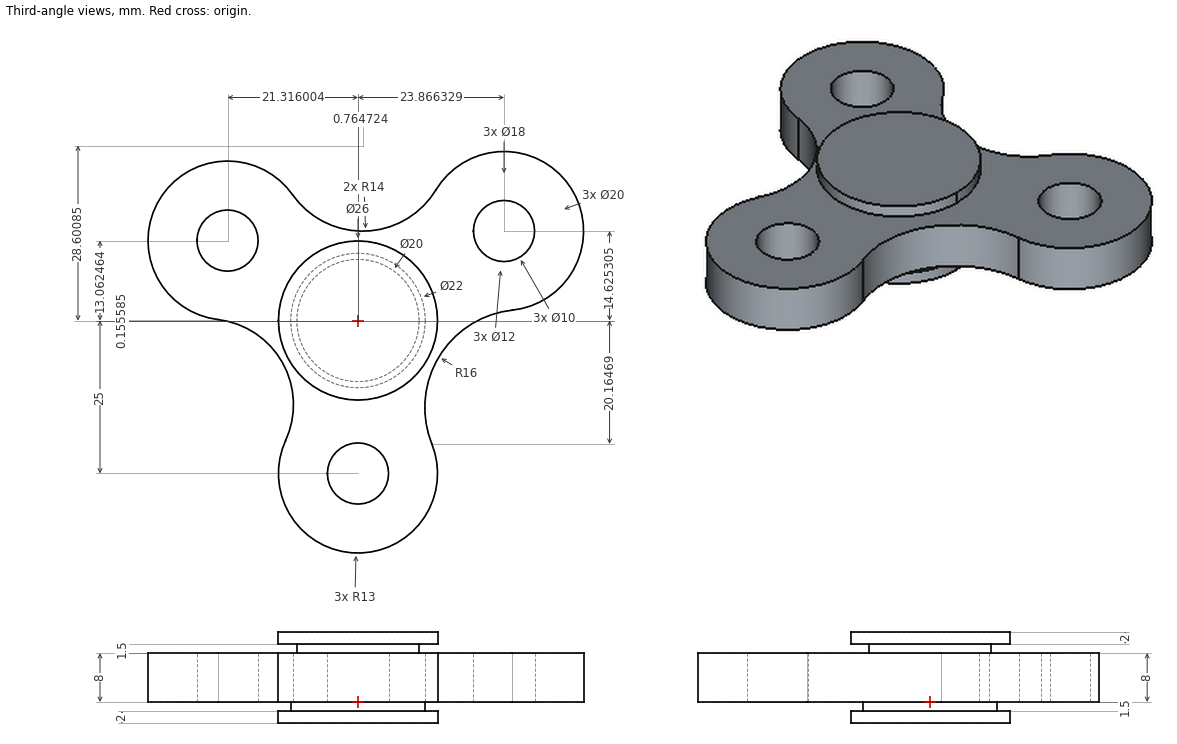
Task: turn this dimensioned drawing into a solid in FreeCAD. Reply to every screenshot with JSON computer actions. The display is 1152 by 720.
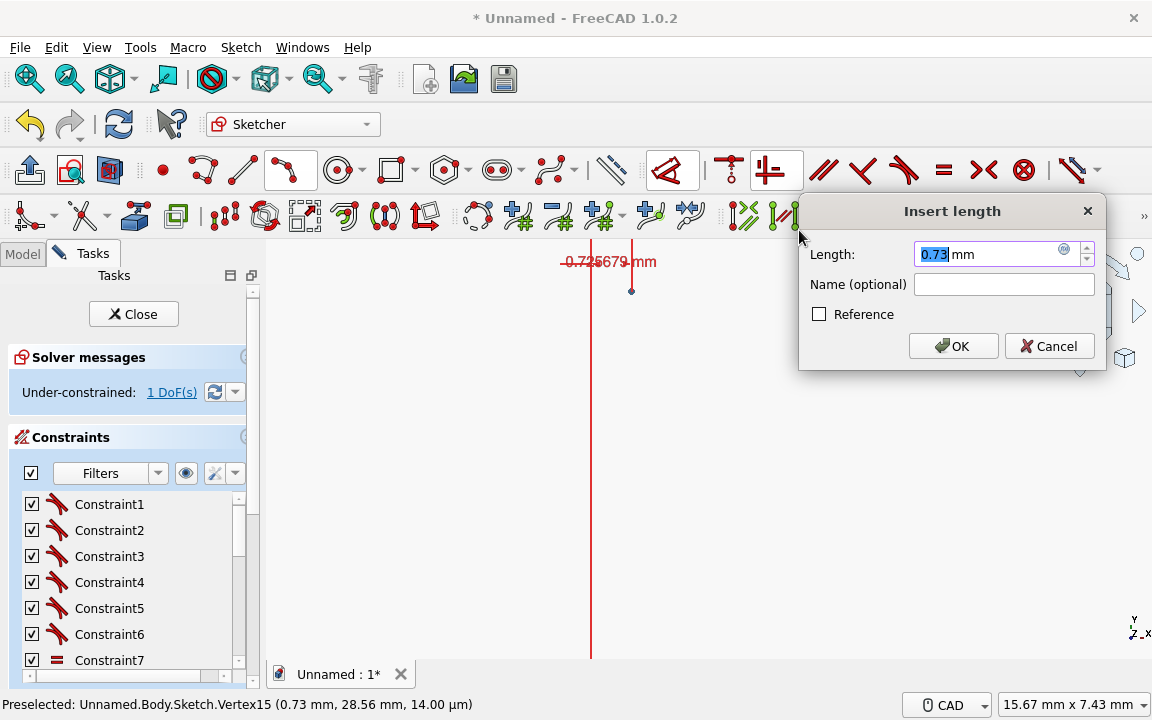
{"action": "type", "text": "0.764724"}
{"action": "key", "text": "Return"}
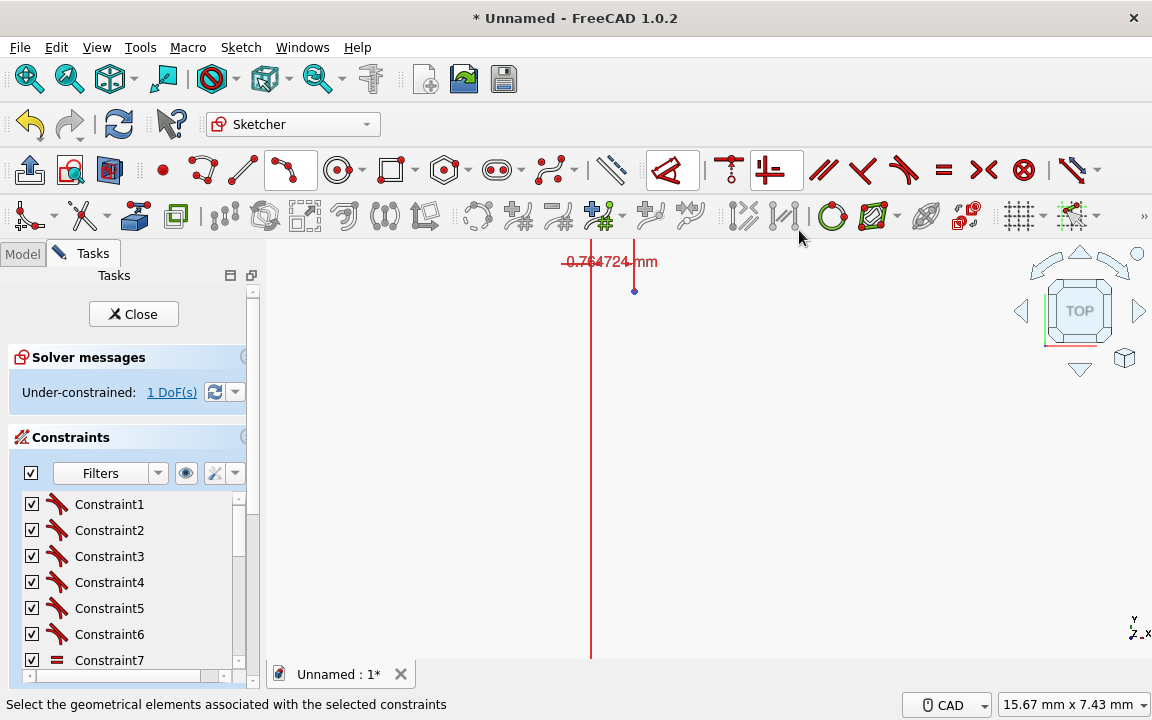
{"action": "scroll", "coordinate": [639, 295], "scroll_direction": "down", "scroll_amount": 13}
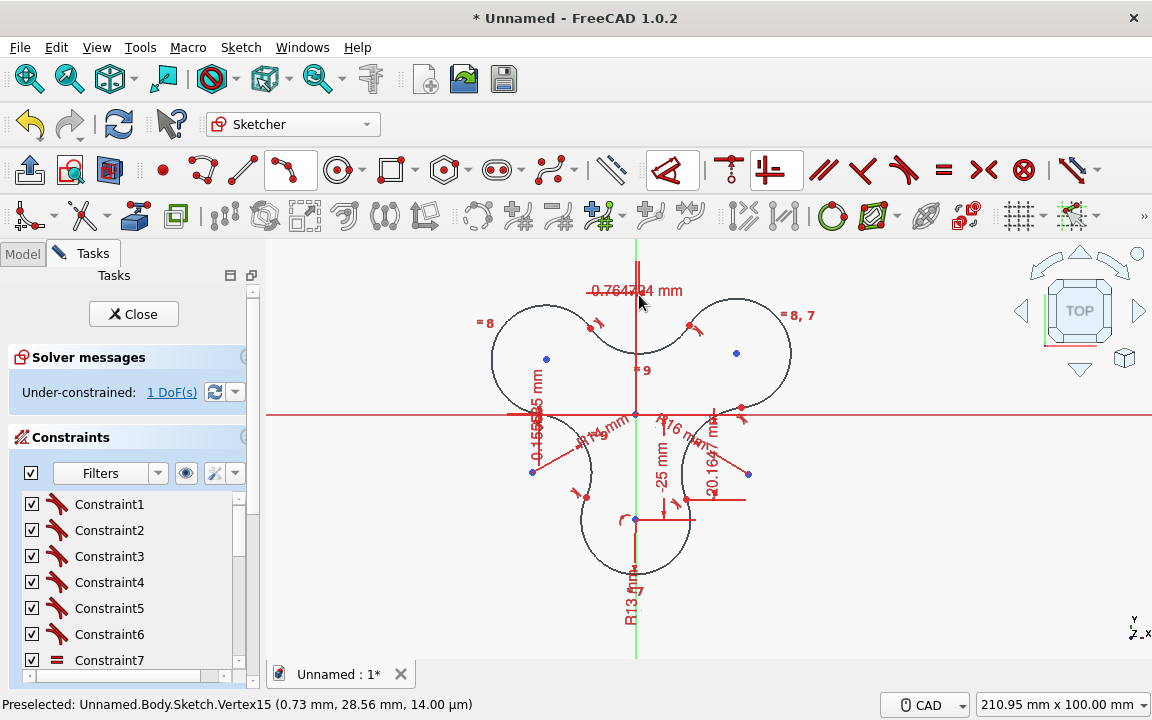
{"action": "left_click", "coordinate": [639, 295]}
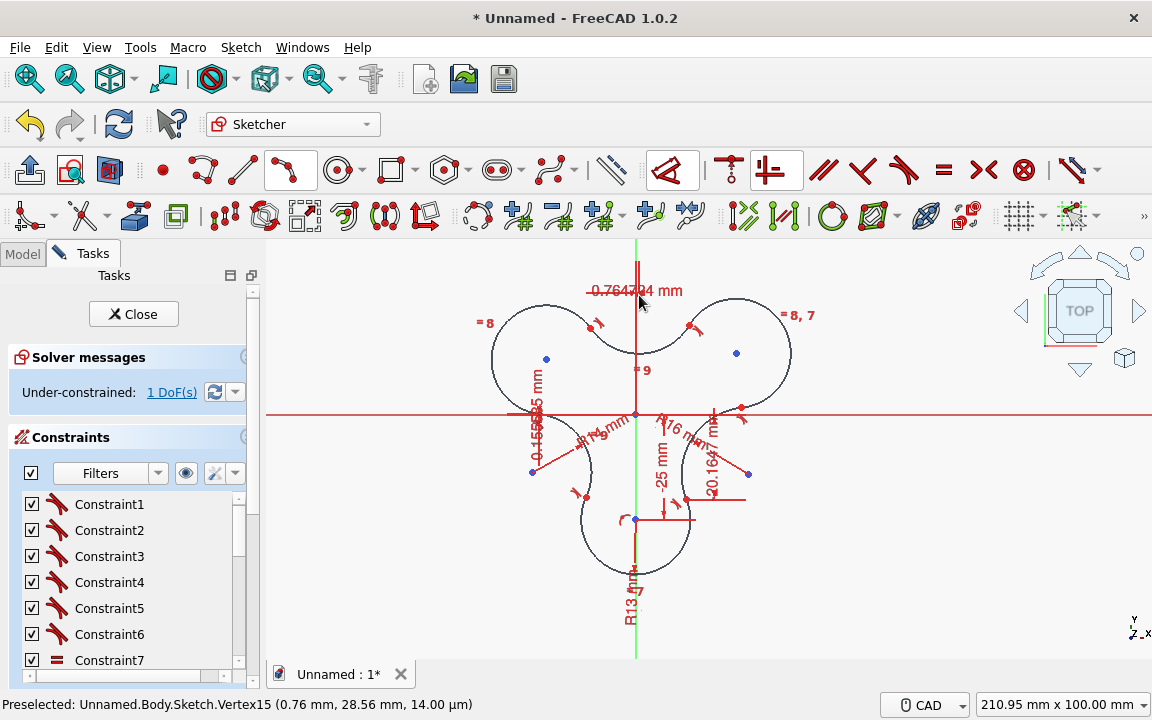
{"action": "key", "text": "i"}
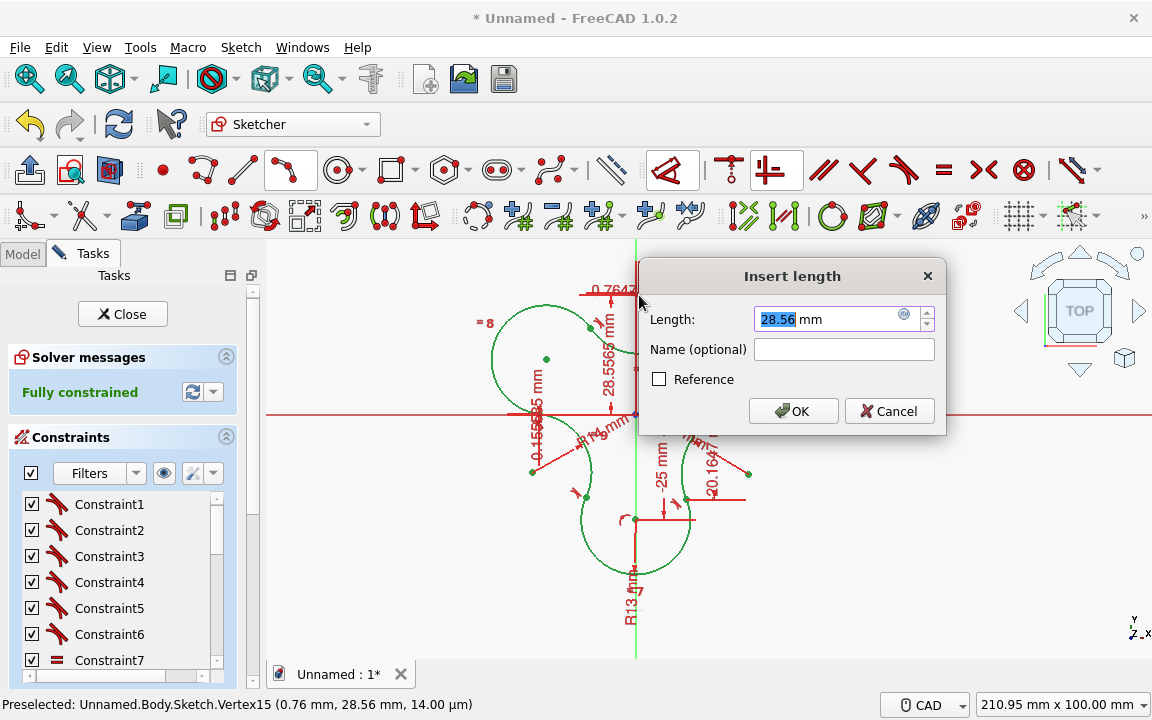
{"action": "type", "text": "28.60085"}
{"action": "key", "text": "Return"}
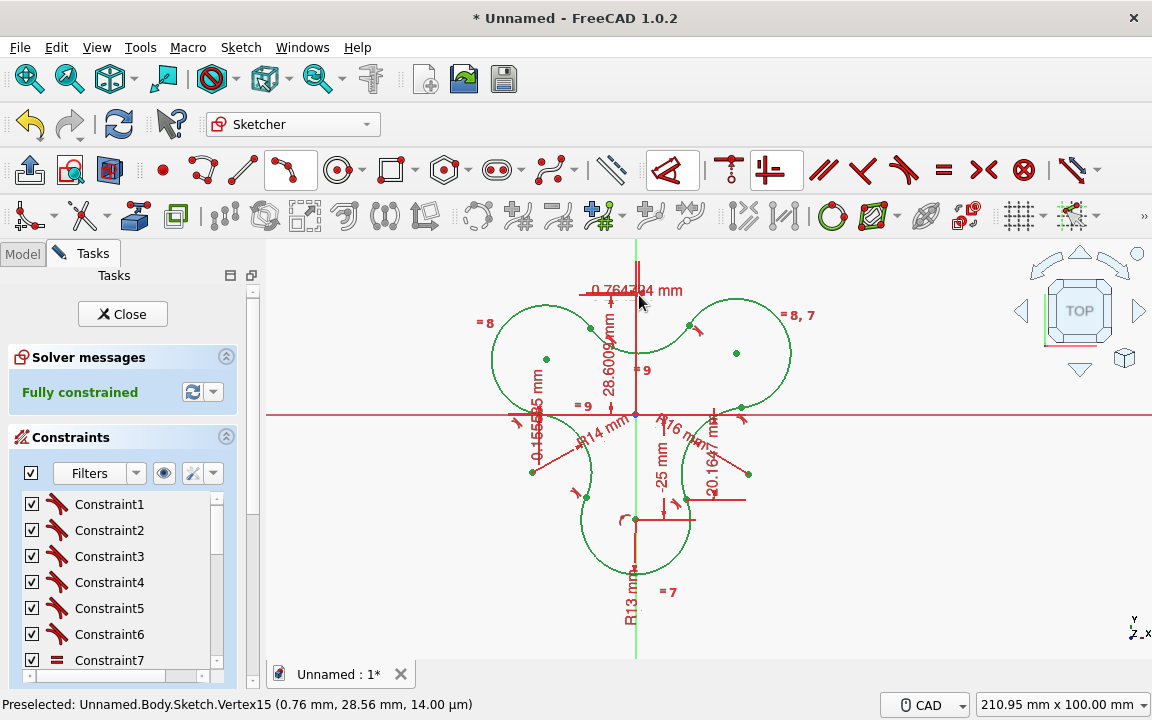
{"action": "left_click", "coordinate": [123, 314]}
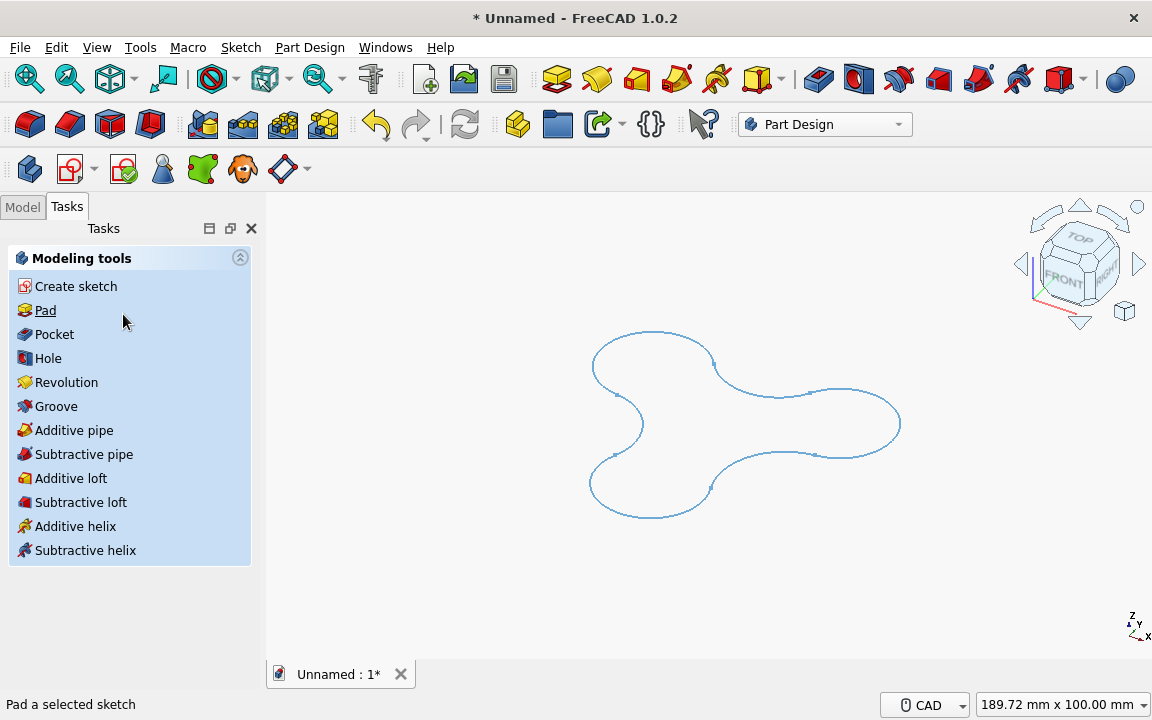
{"action": "left_click", "coordinate": [558, 80]}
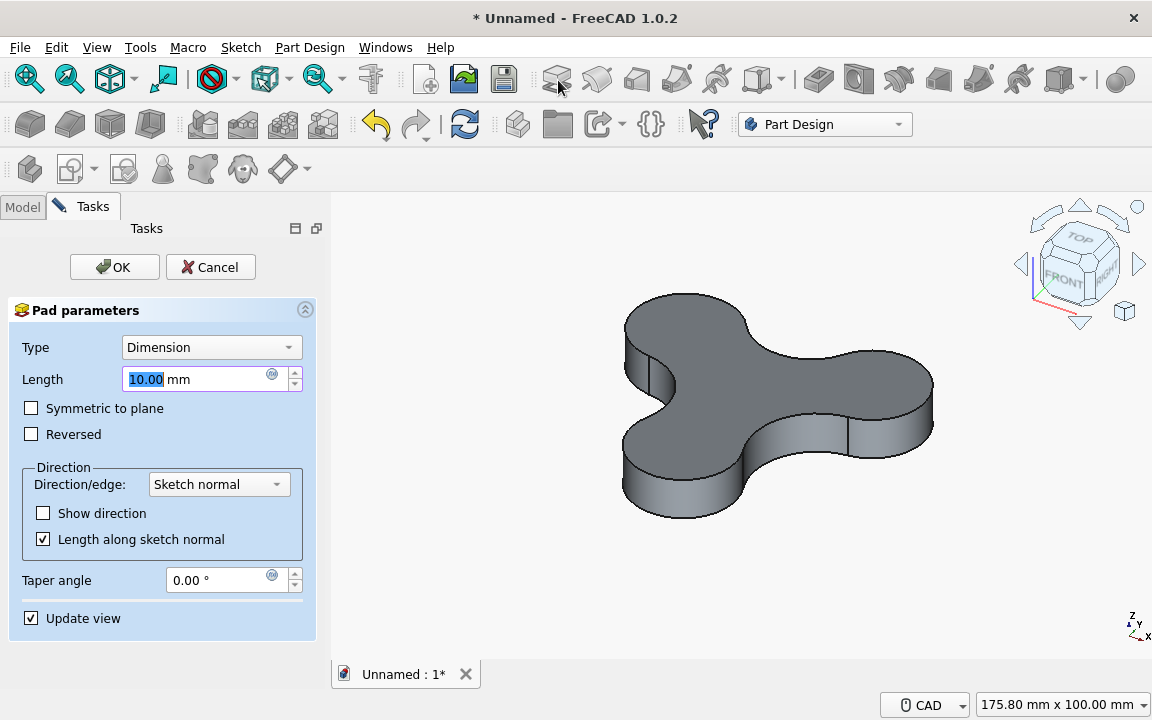
{"action": "type", "text": "8"}
{"action": "key", "text": "Tab"}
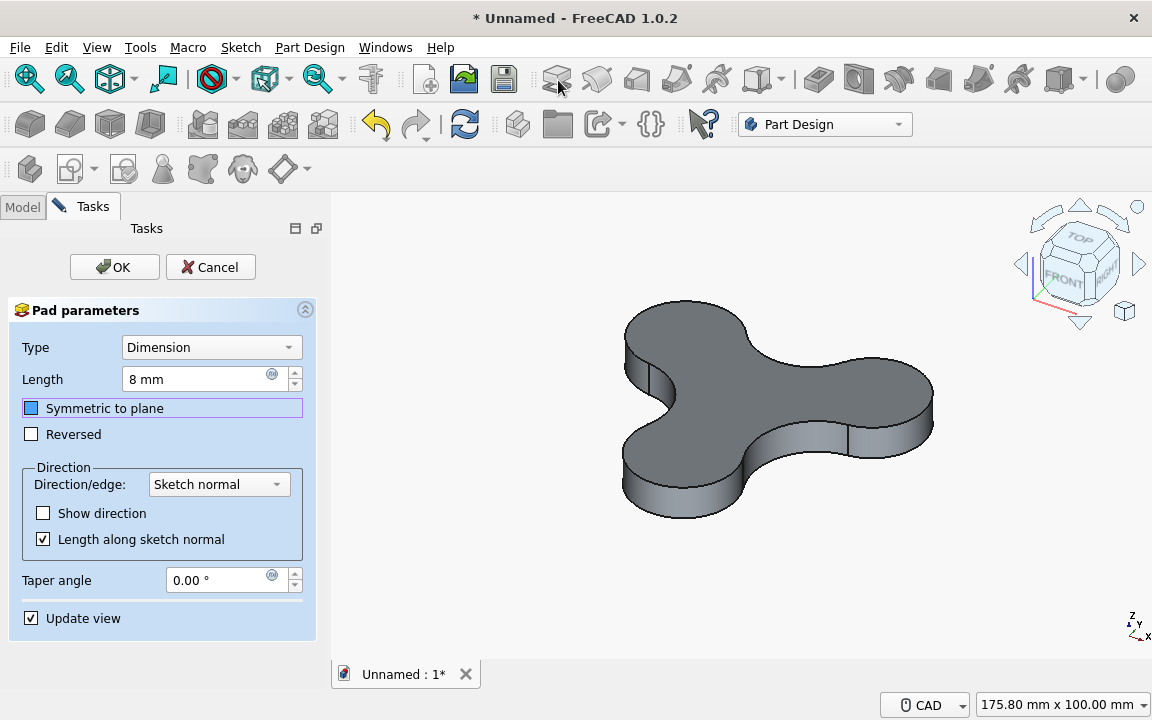
{"action": "left_click", "coordinate": [115, 267]}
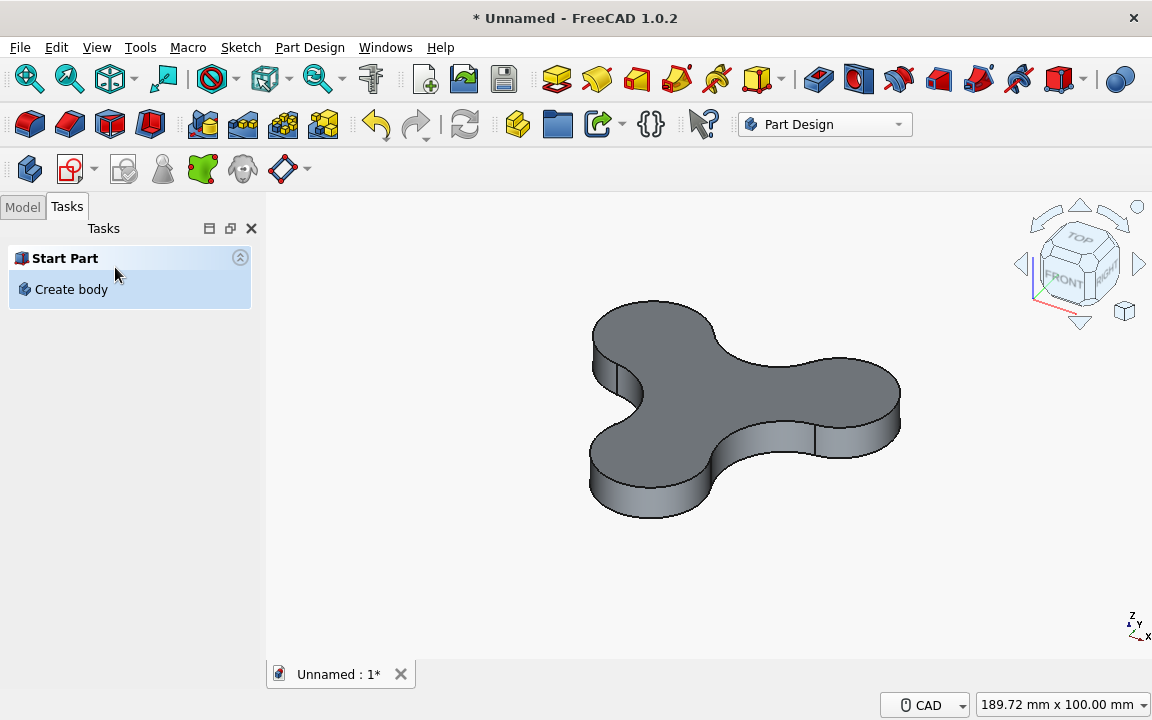
{"action": "left_click", "coordinate": [828, 391]}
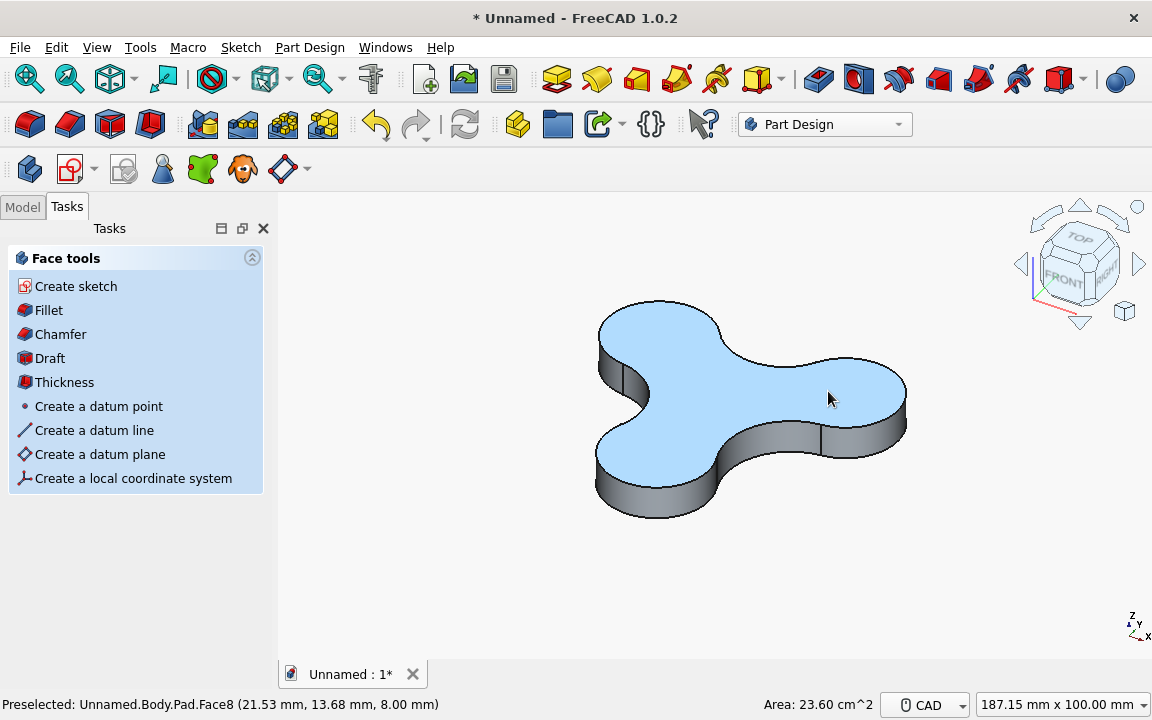
{"action": "left_click", "coordinate": [70, 170]}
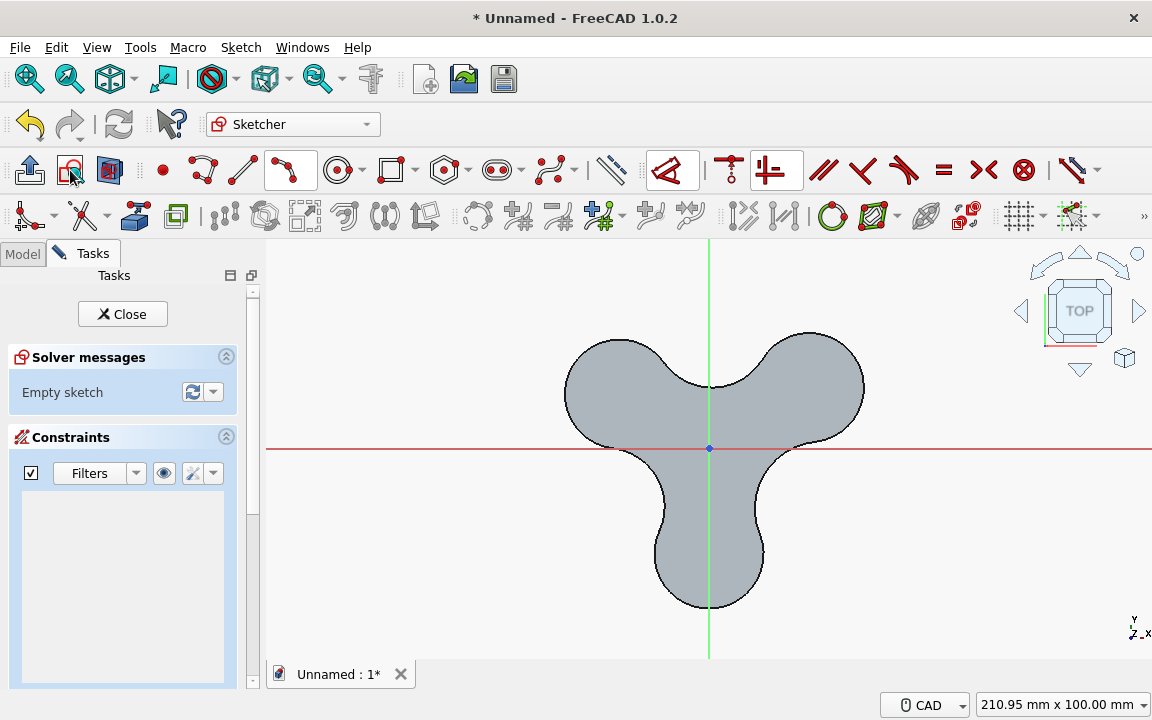
{"action": "scroll", "coordinate": [739, 449], "scroll_direction": "up", "scroll_amount": 6}